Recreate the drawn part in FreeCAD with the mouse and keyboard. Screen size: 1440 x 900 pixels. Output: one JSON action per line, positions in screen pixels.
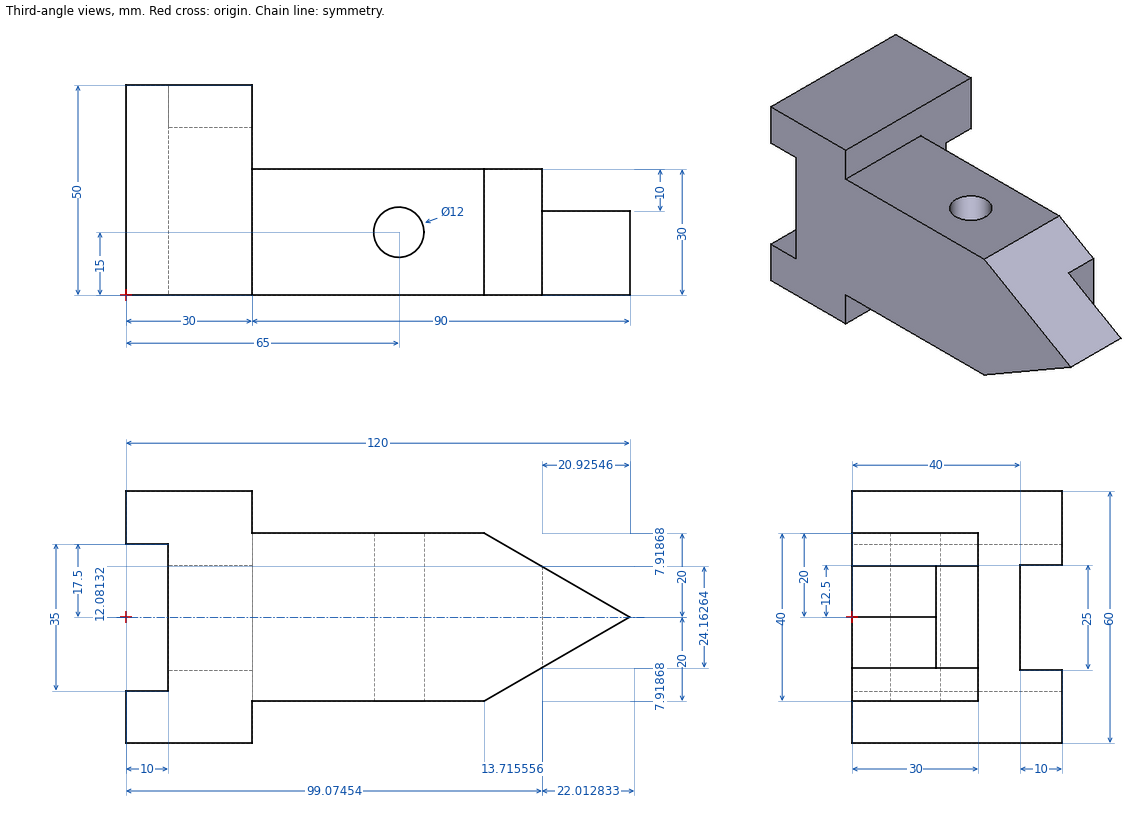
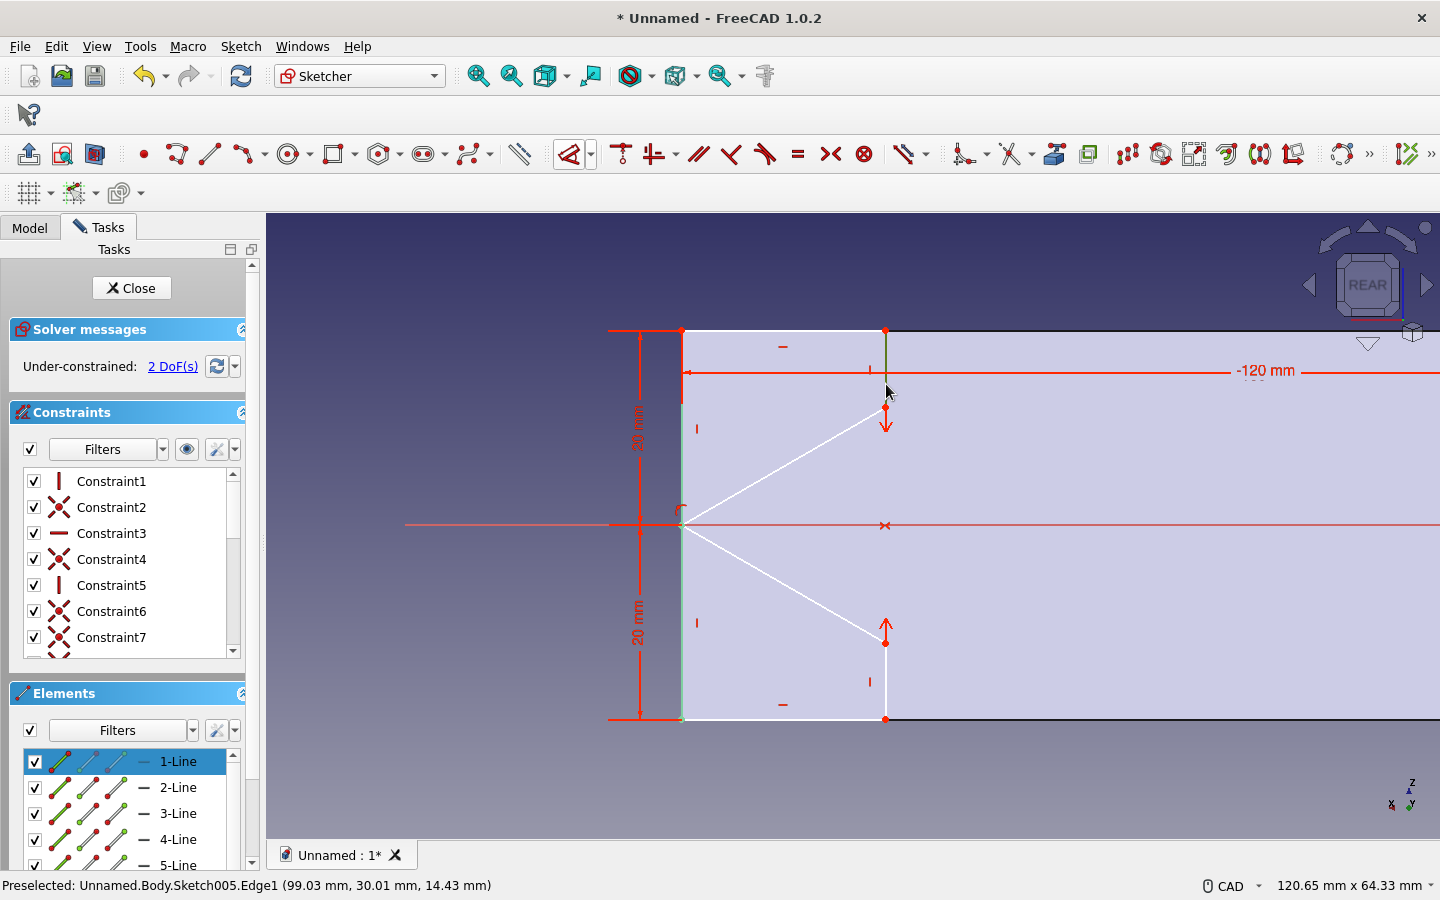
{"action": "key", "text": "i"}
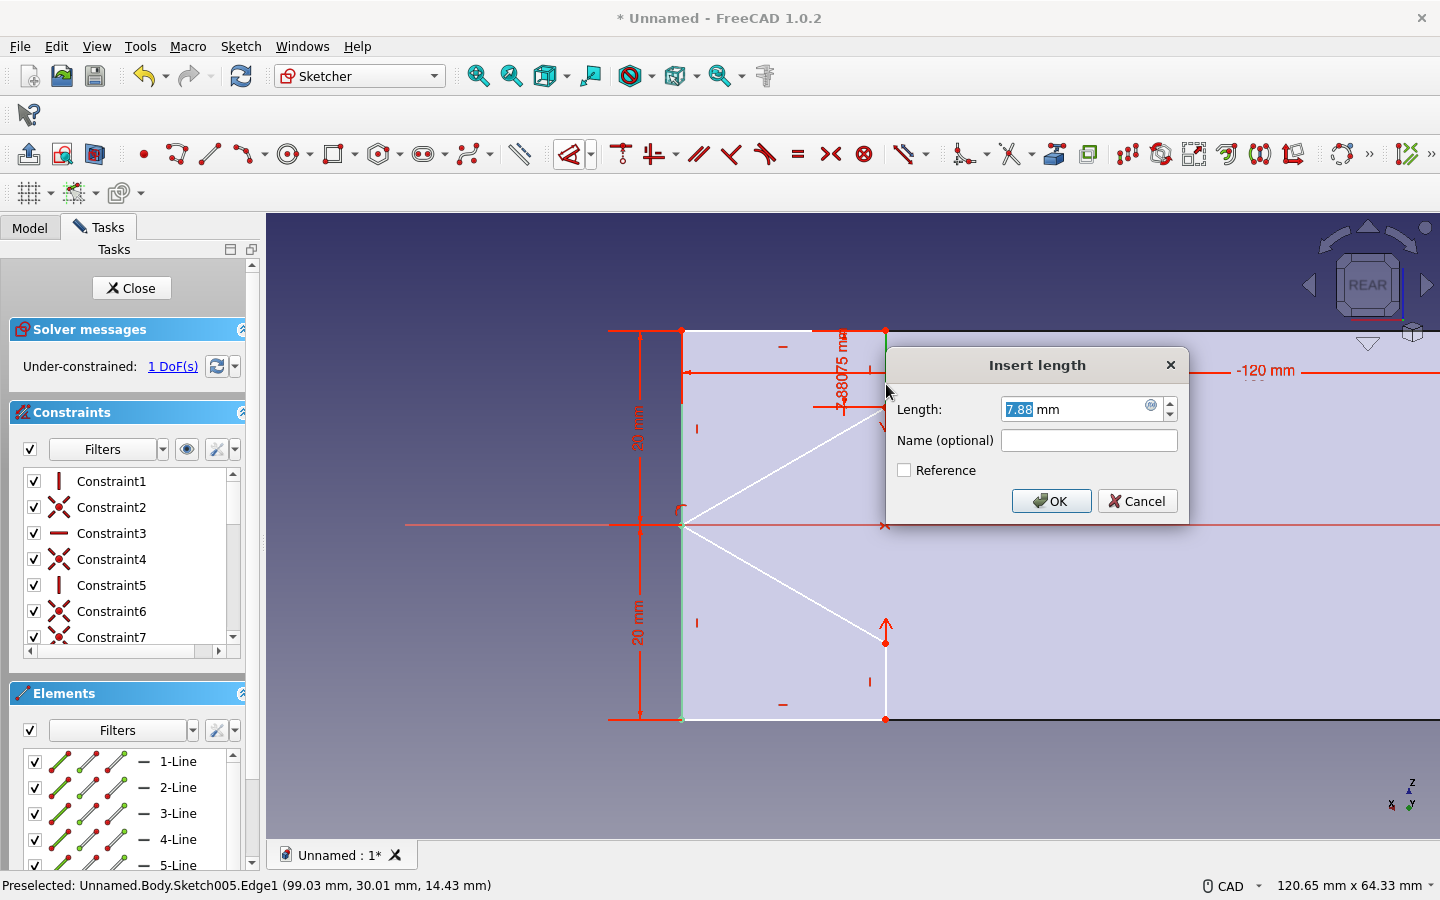
{"action": "type", "text": "7.91868"}
{"action": "key", "text": "Return"}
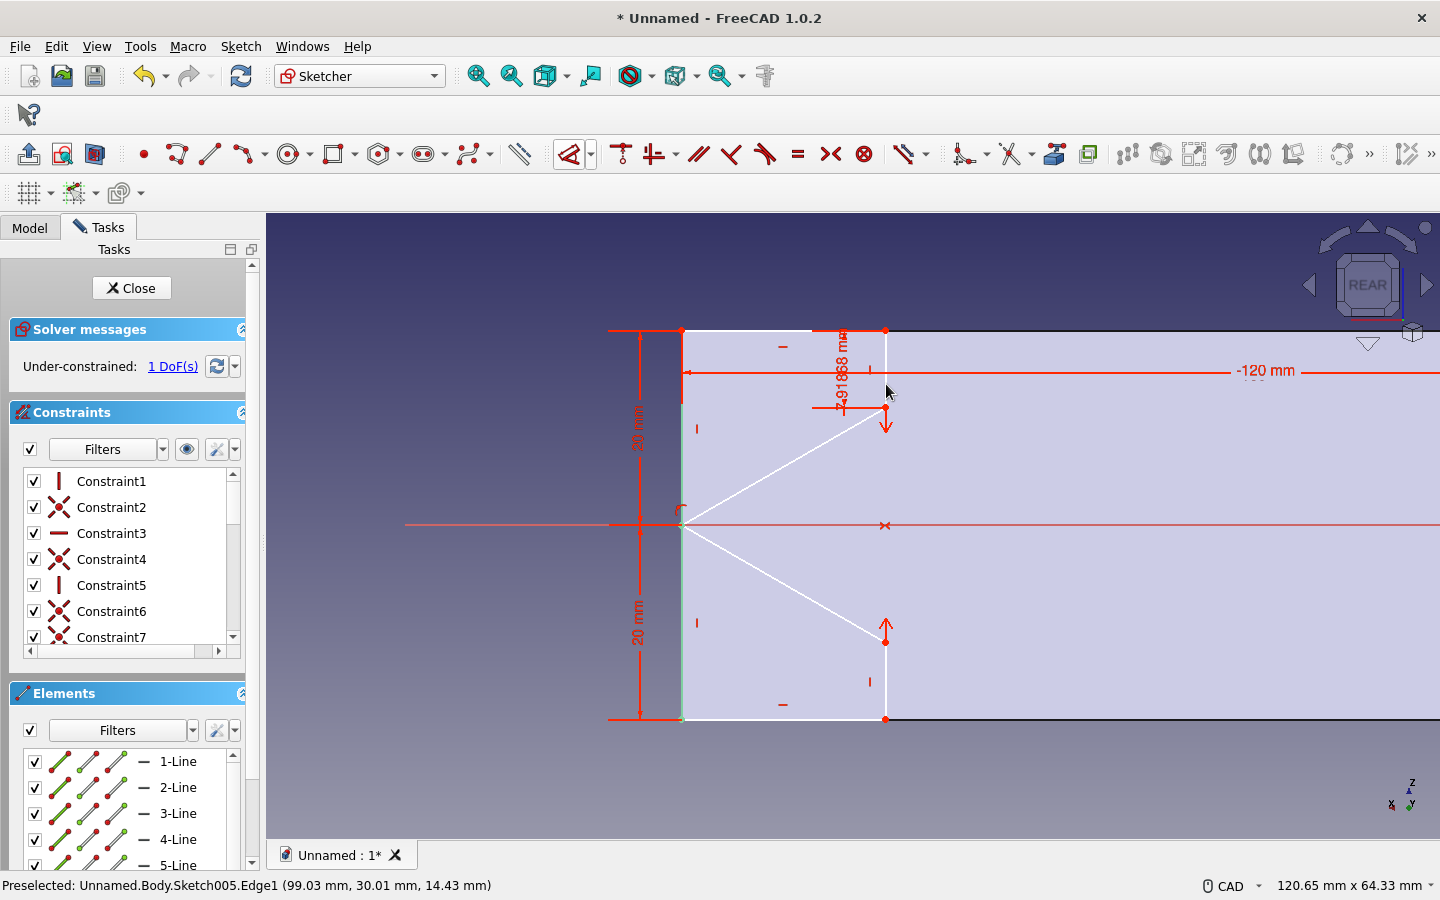
{"action": "left_click", "coordinate": [825, 331]}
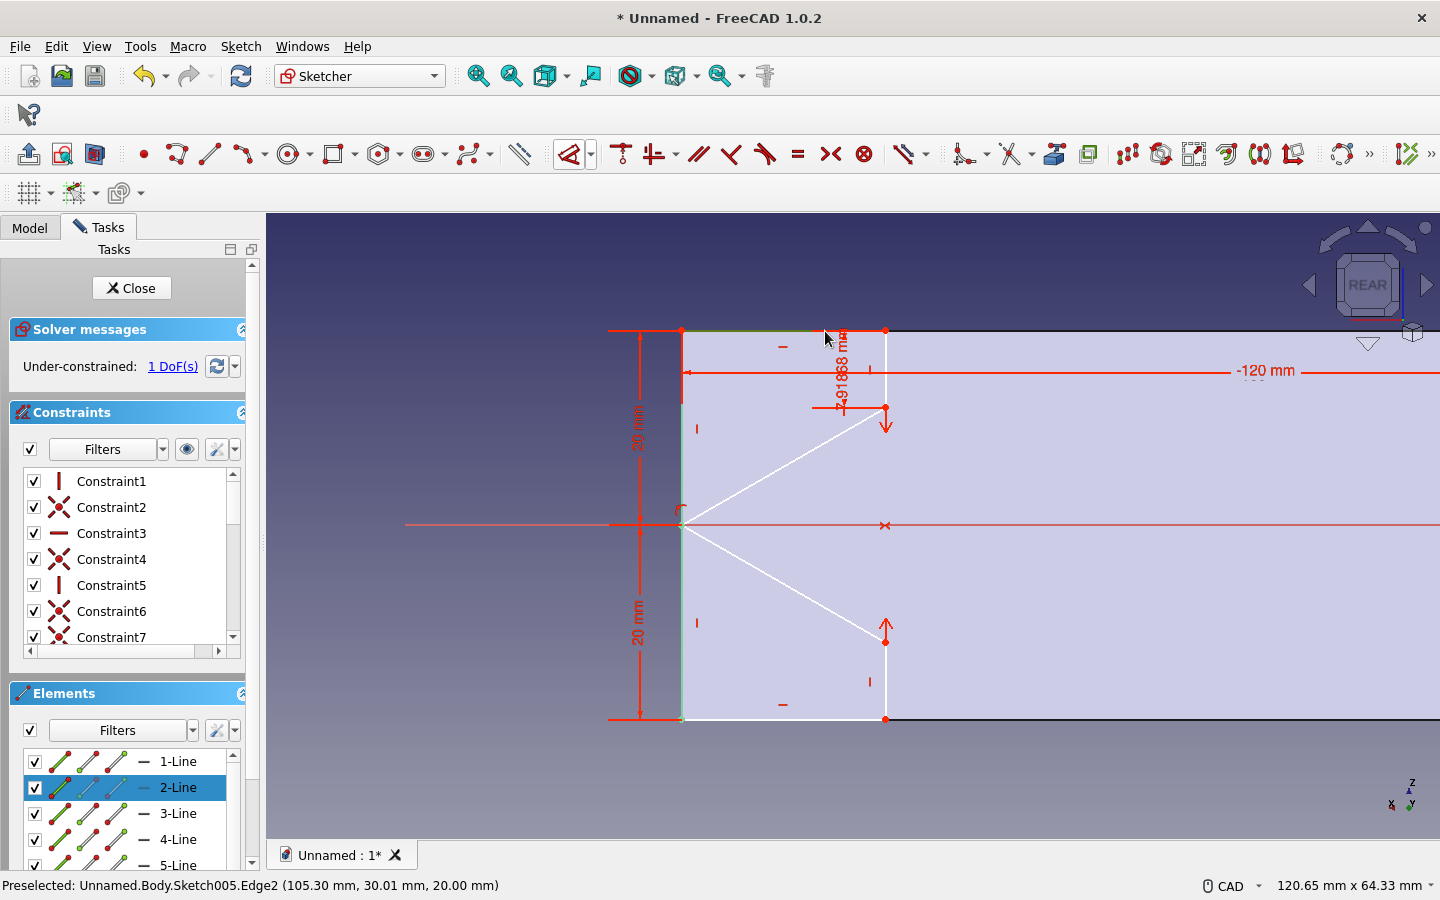
{"action": "key", "text": "l"}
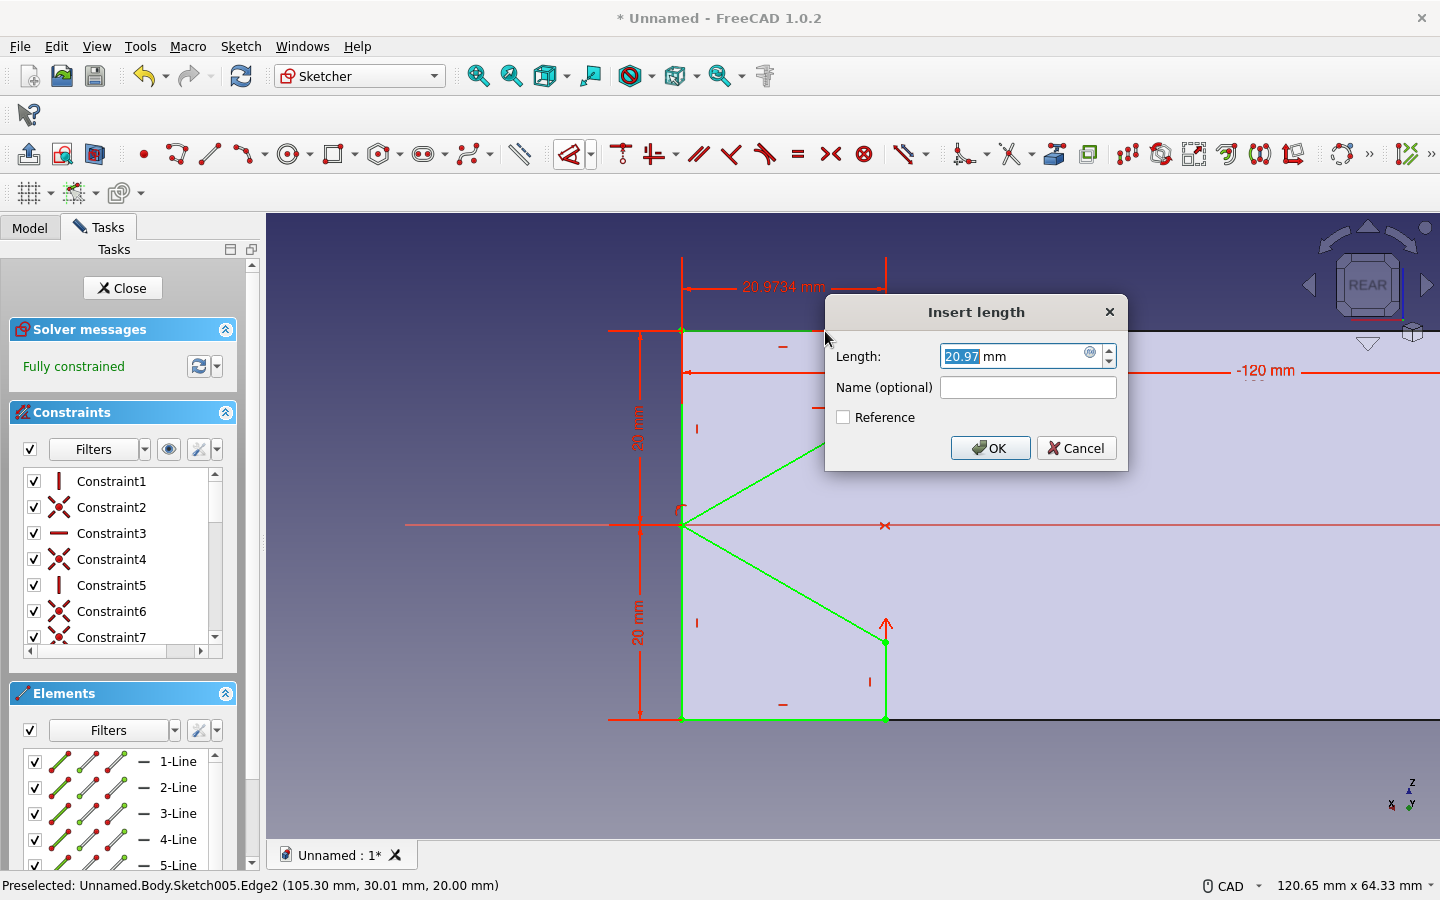
{"action": "type", "text": "20.92546"}
{"action": "key", "text": "Return"}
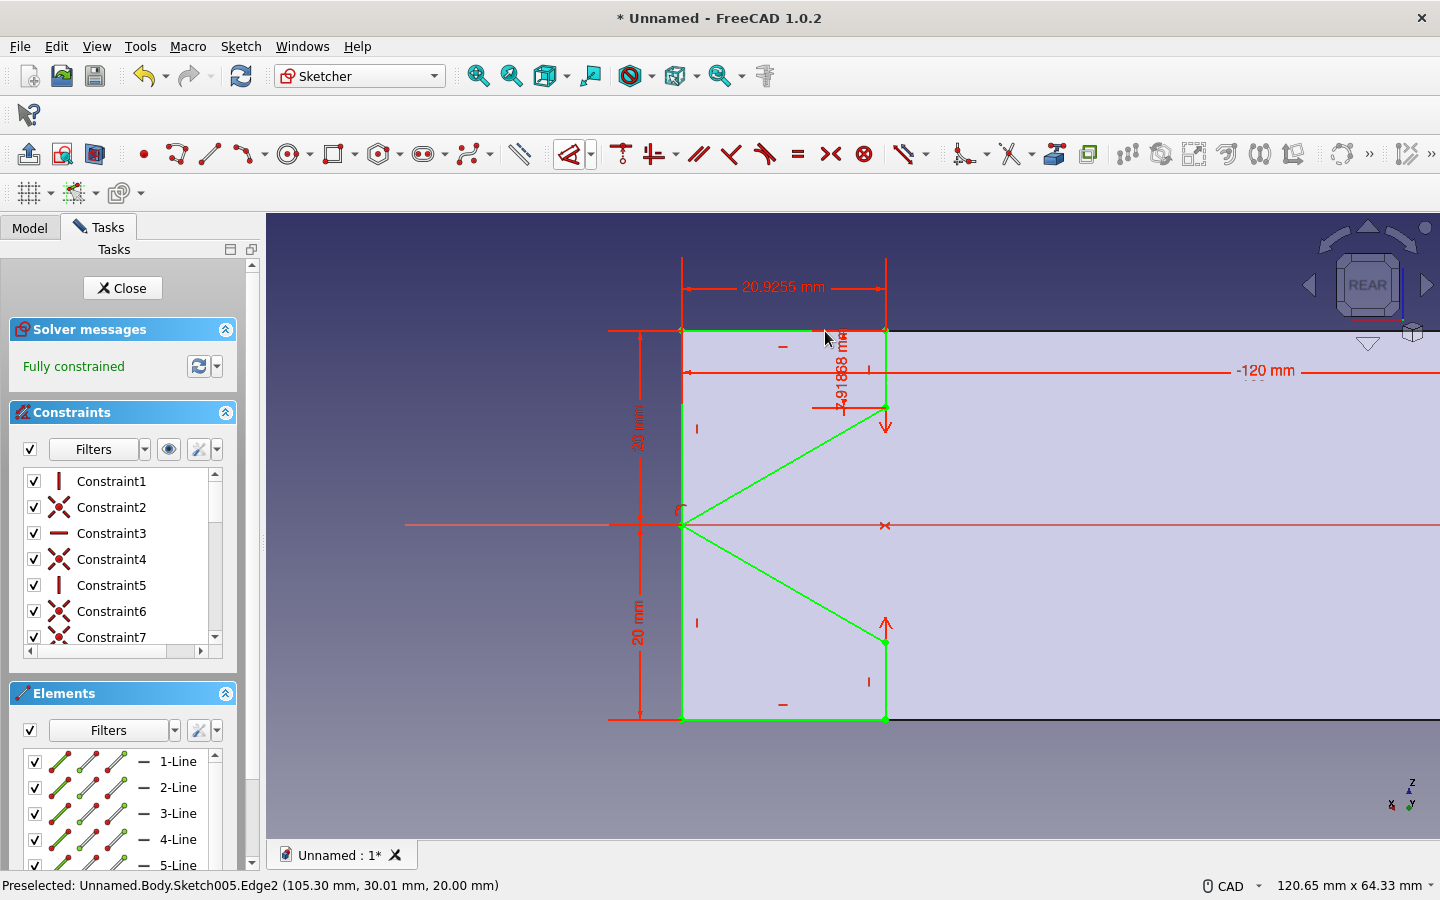
{"action": "left_click", "coordinate": [123, 288]}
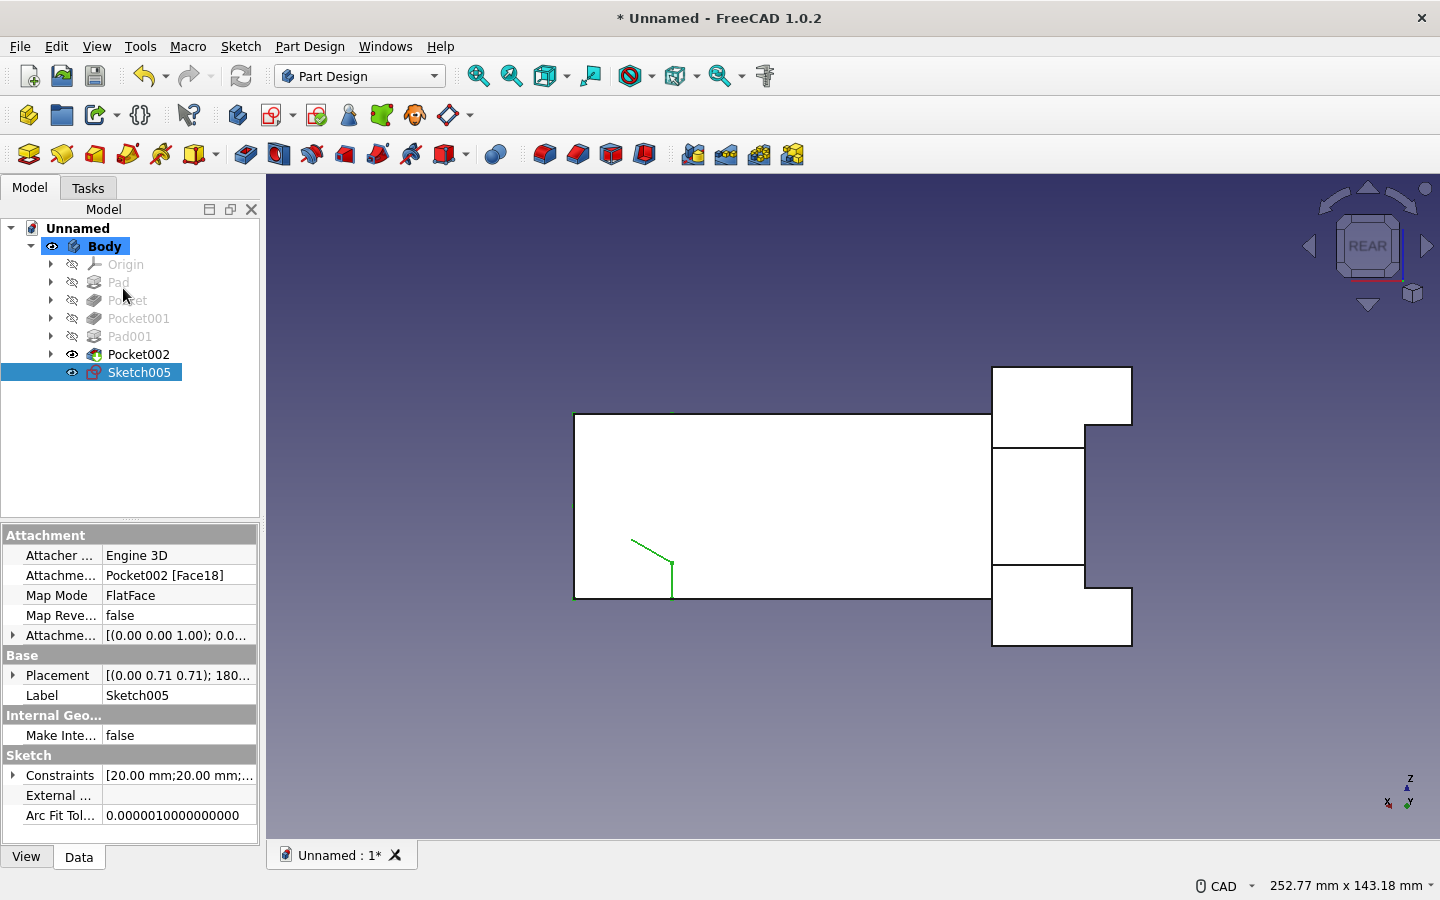
{"action": "left_click", "coordinate": [246, 154]}